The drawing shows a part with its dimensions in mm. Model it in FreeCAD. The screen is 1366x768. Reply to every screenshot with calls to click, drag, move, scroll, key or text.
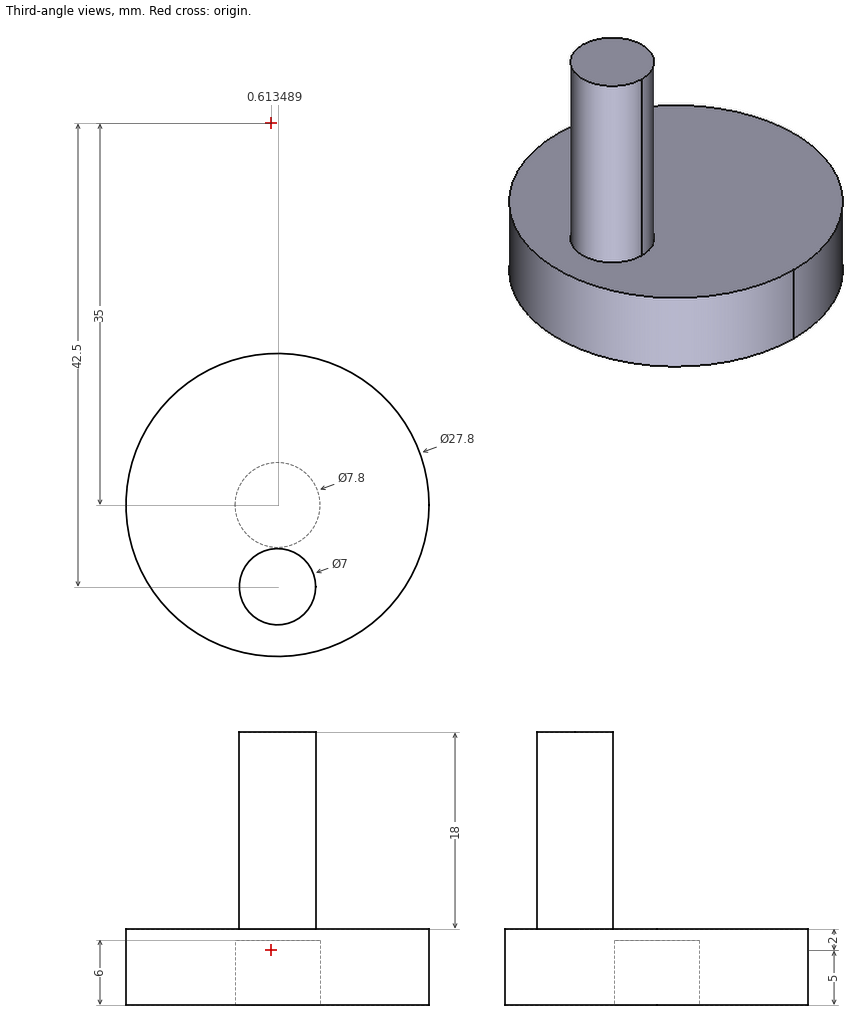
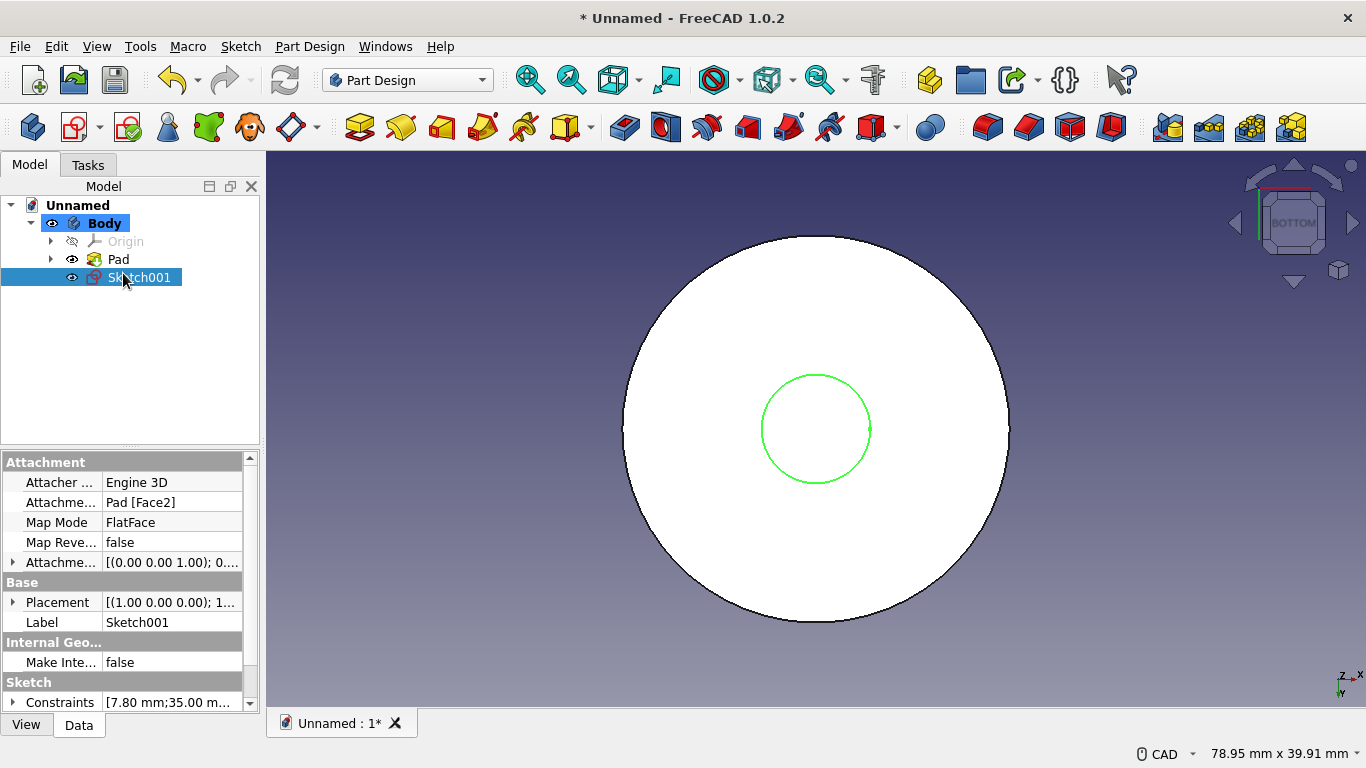
click(625, 128)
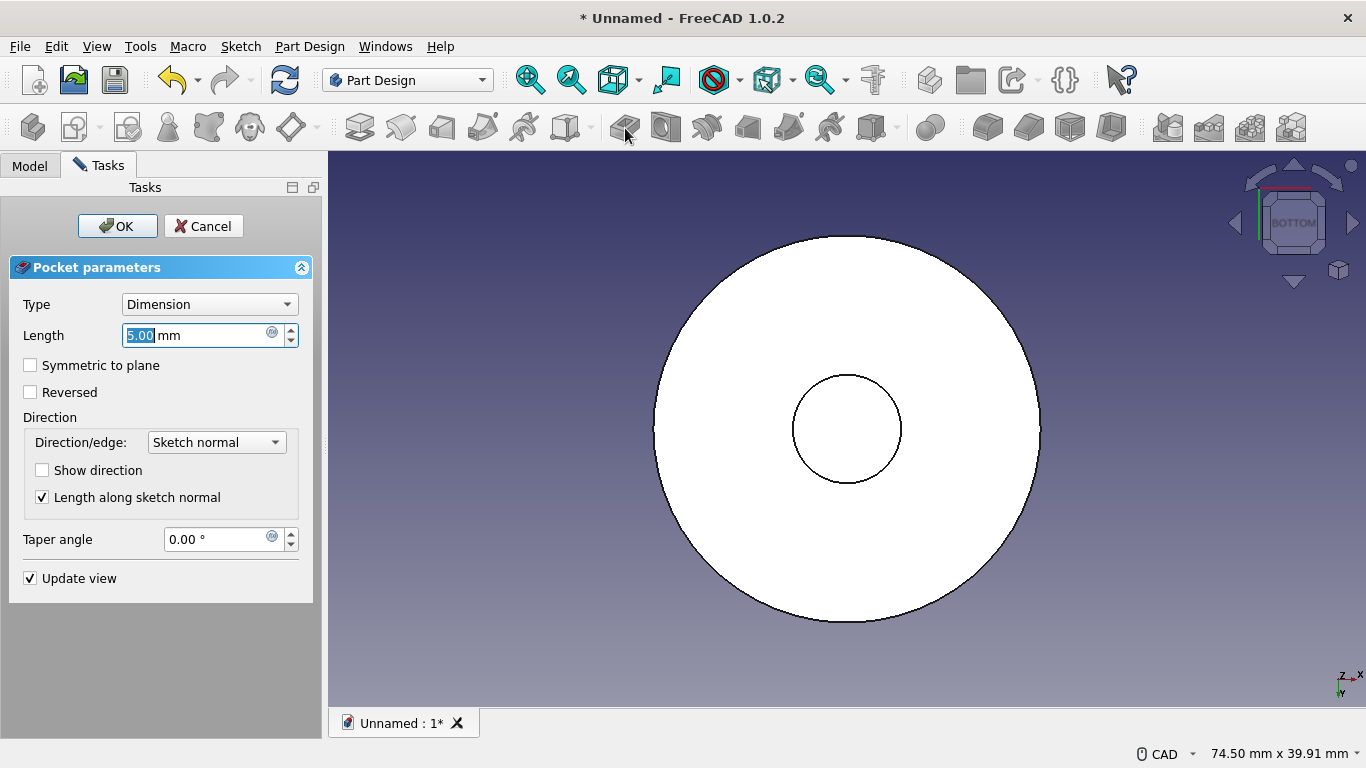
text(6)
key(Tab)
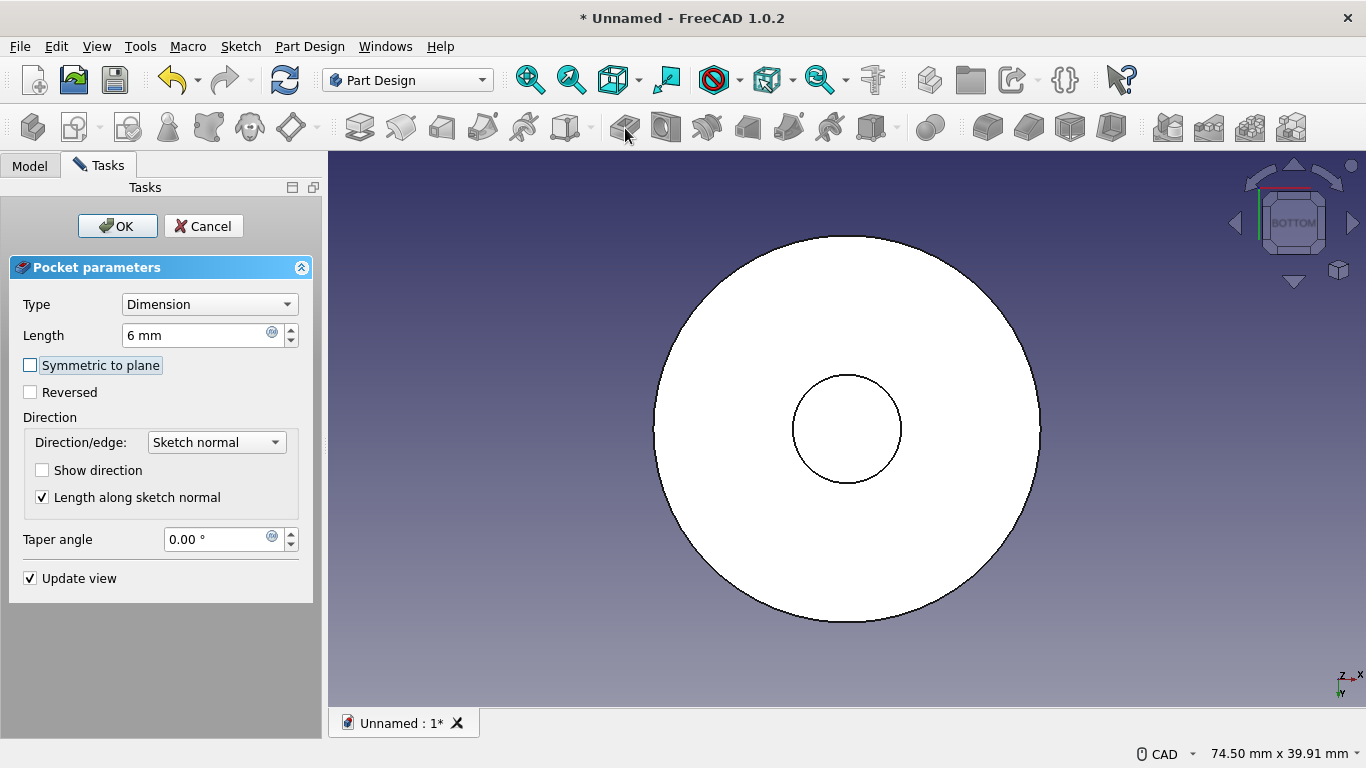
click(118, 226)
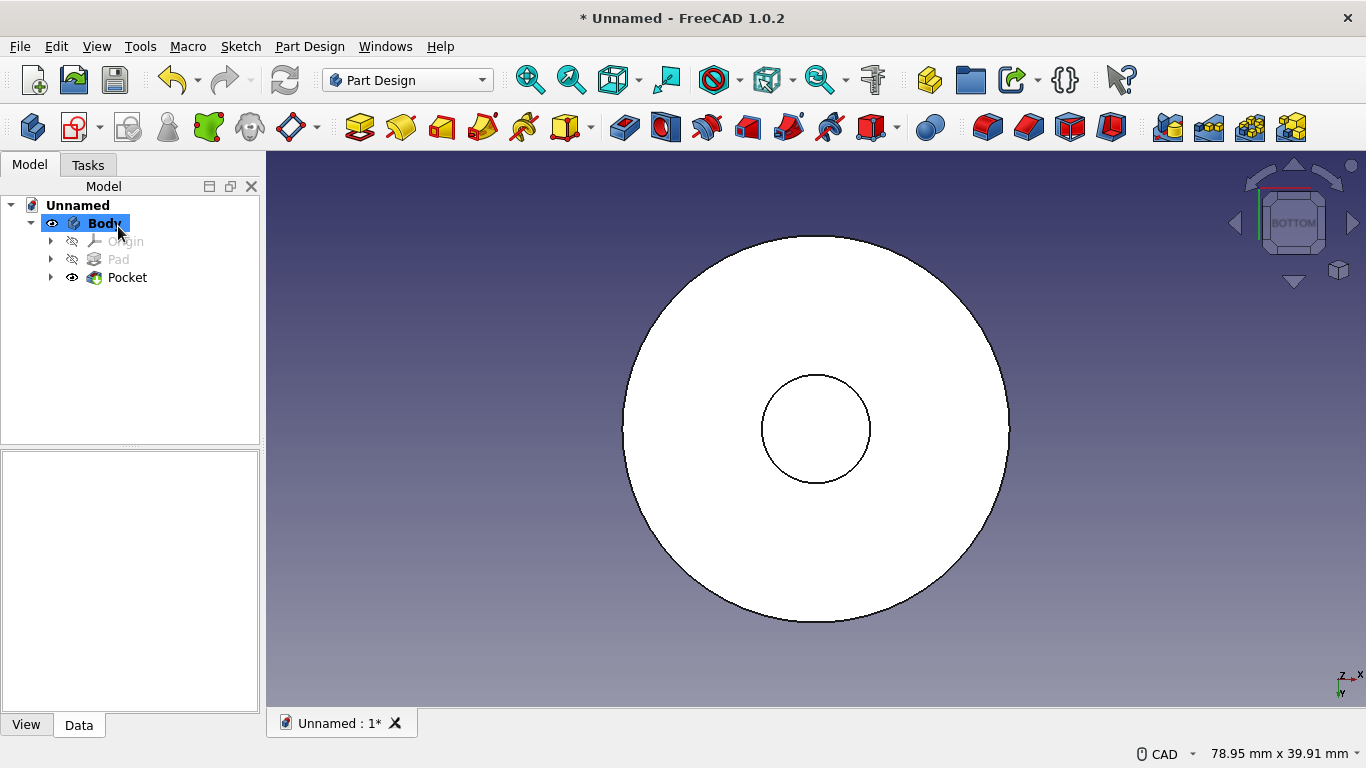
key(0)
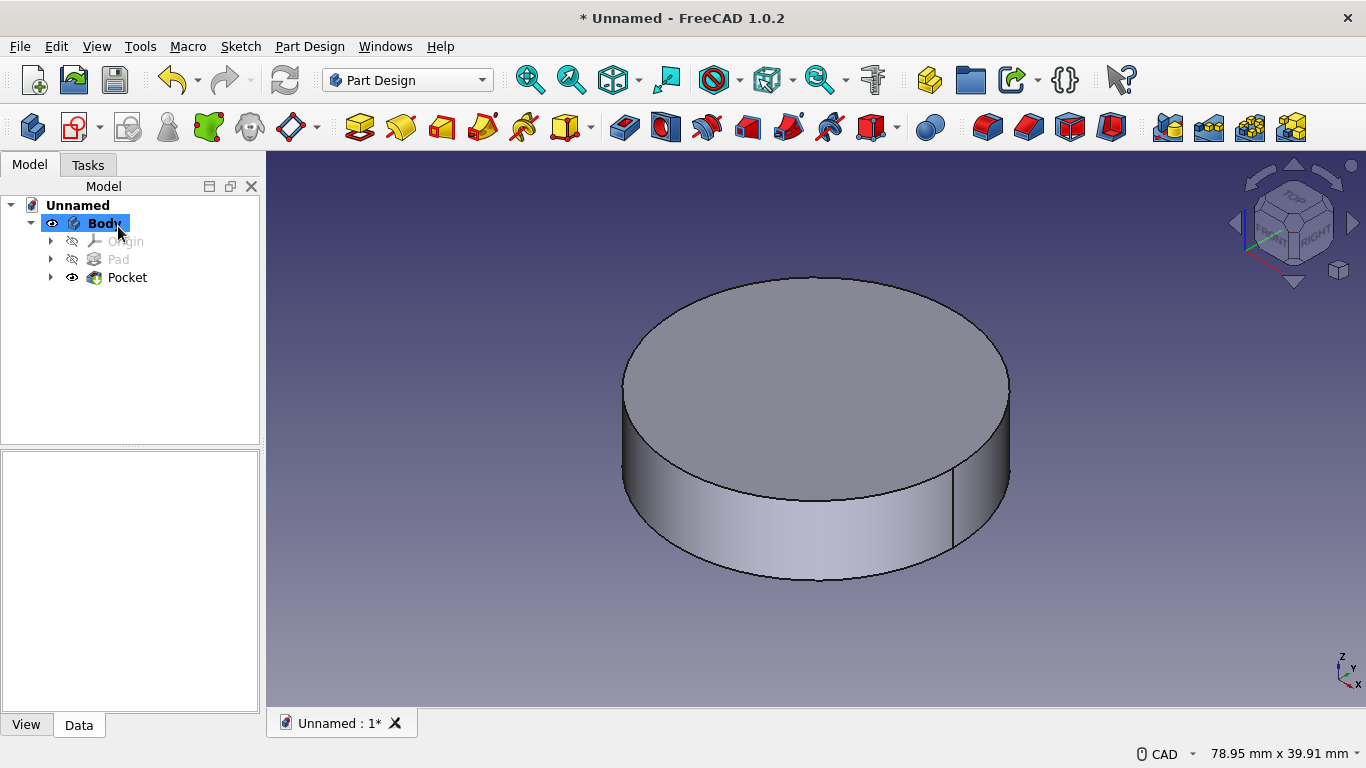
click(816, 388)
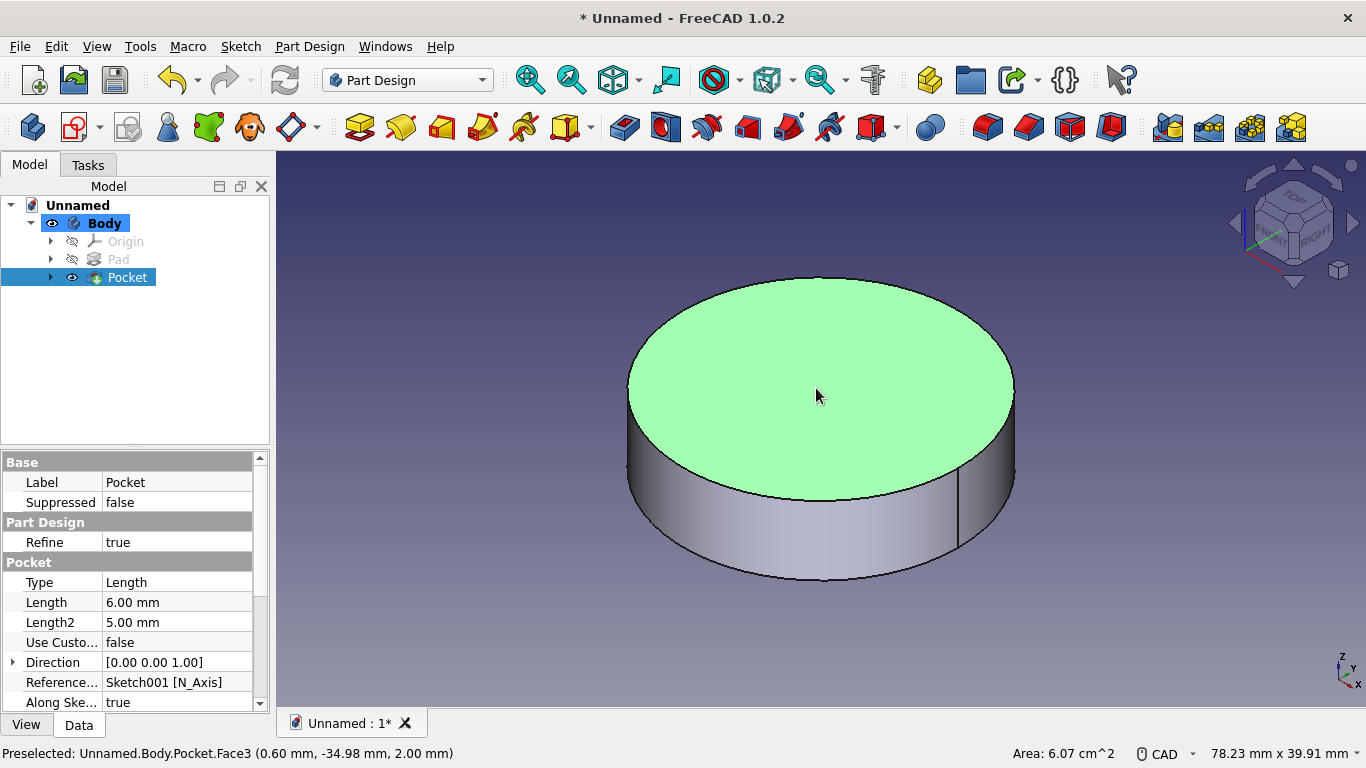
click(74, 128)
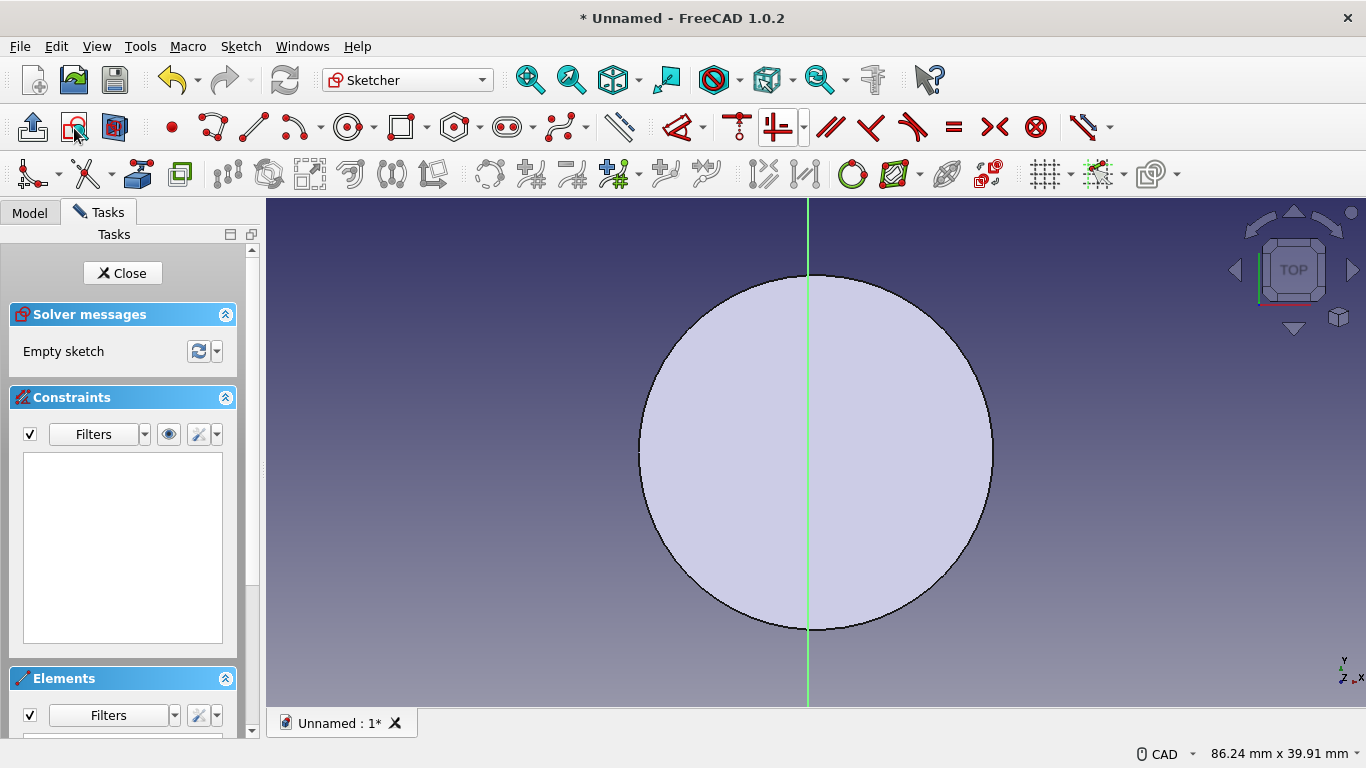
scroll(846, 589, up, 6)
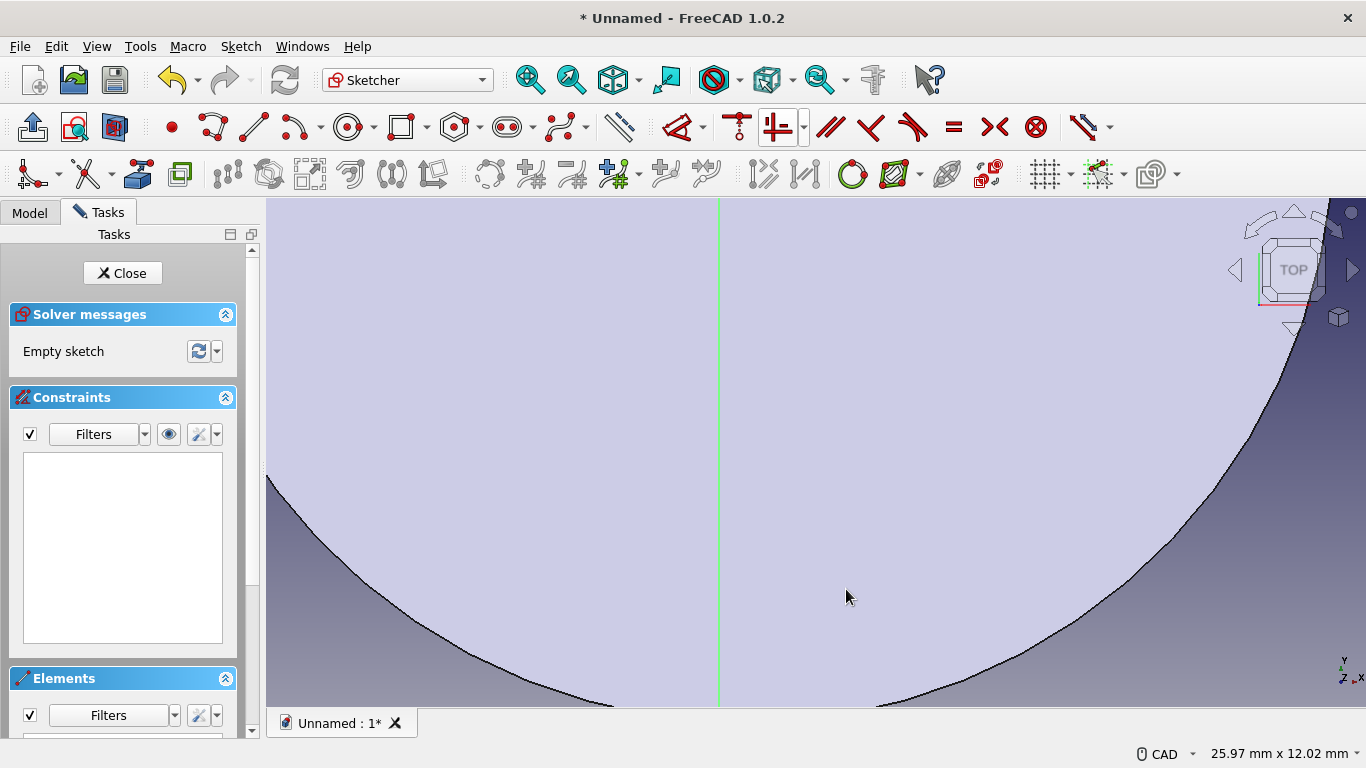
click(348, 128)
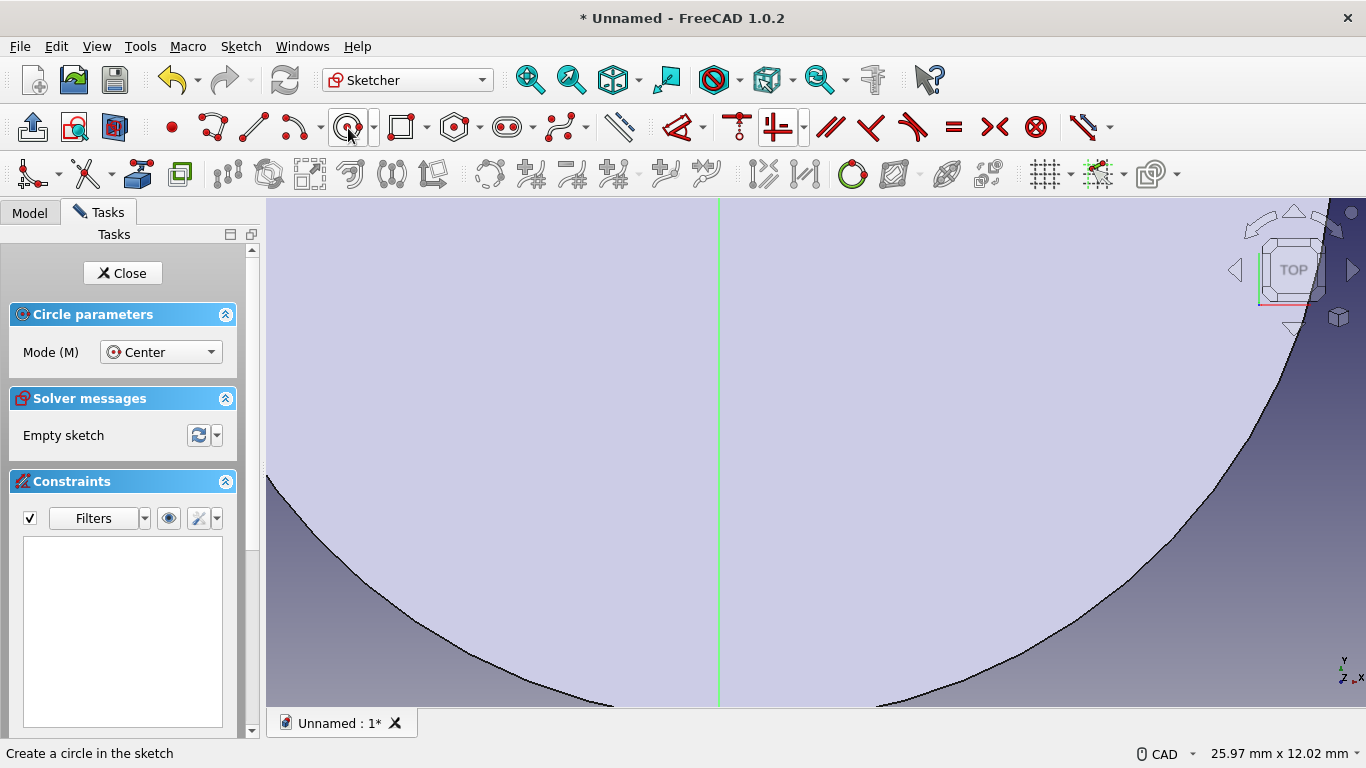
click(745, 452)
move(850, 347)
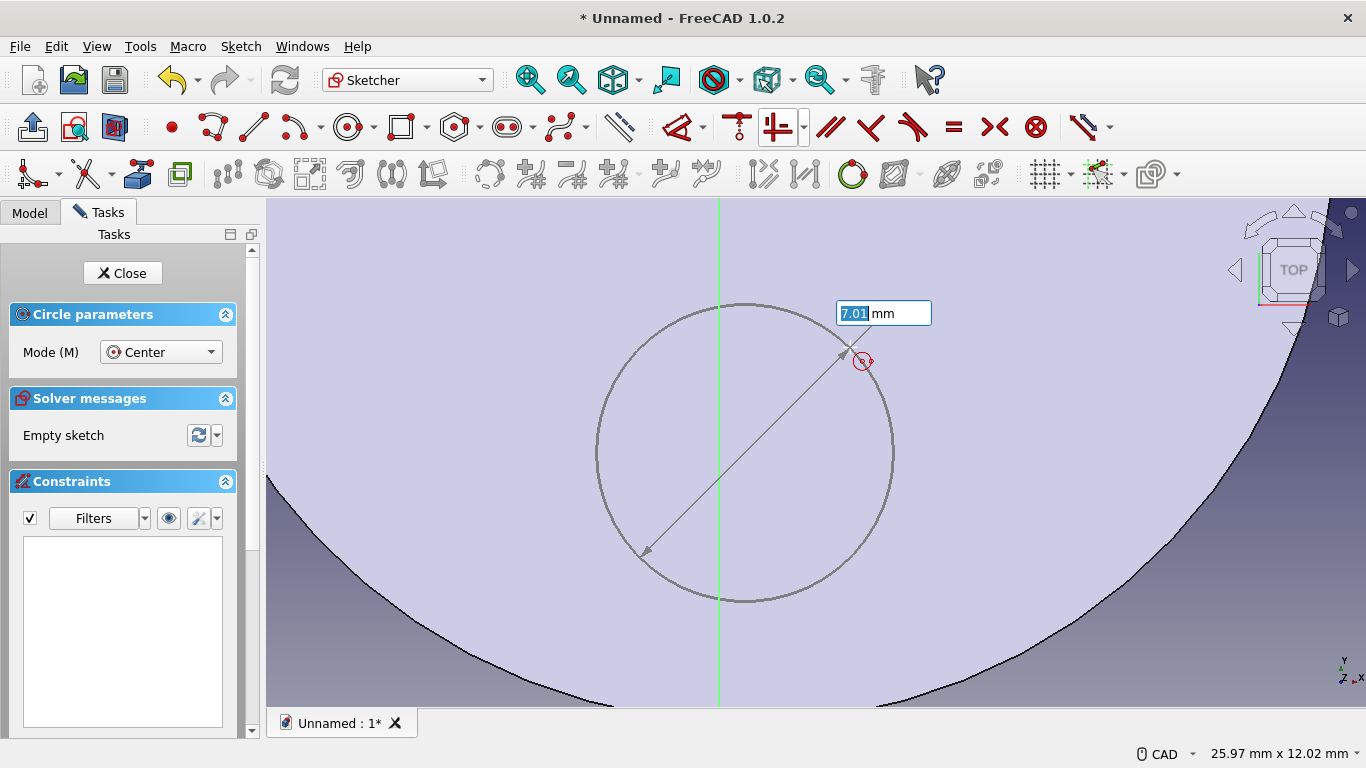
text(7)
key(Return)
key(Escape)